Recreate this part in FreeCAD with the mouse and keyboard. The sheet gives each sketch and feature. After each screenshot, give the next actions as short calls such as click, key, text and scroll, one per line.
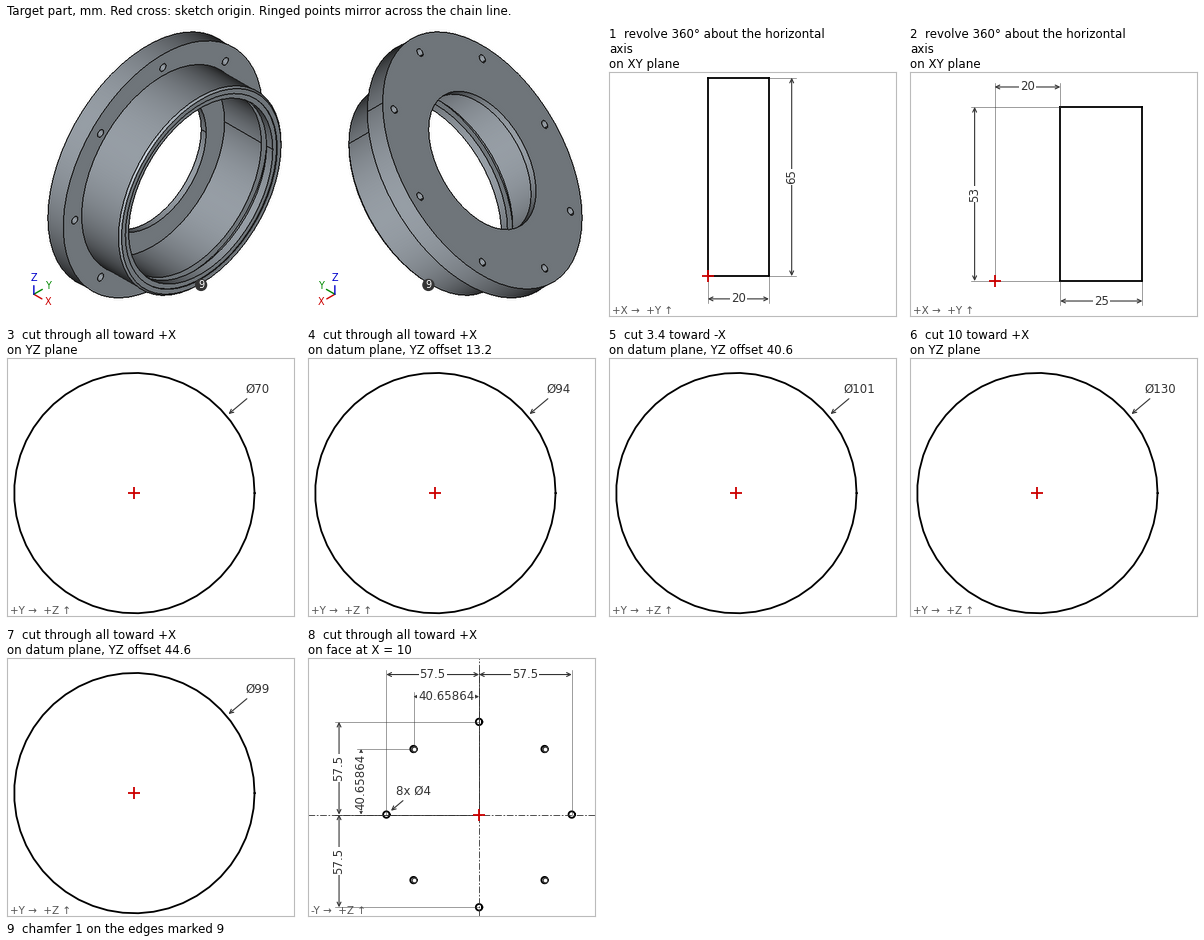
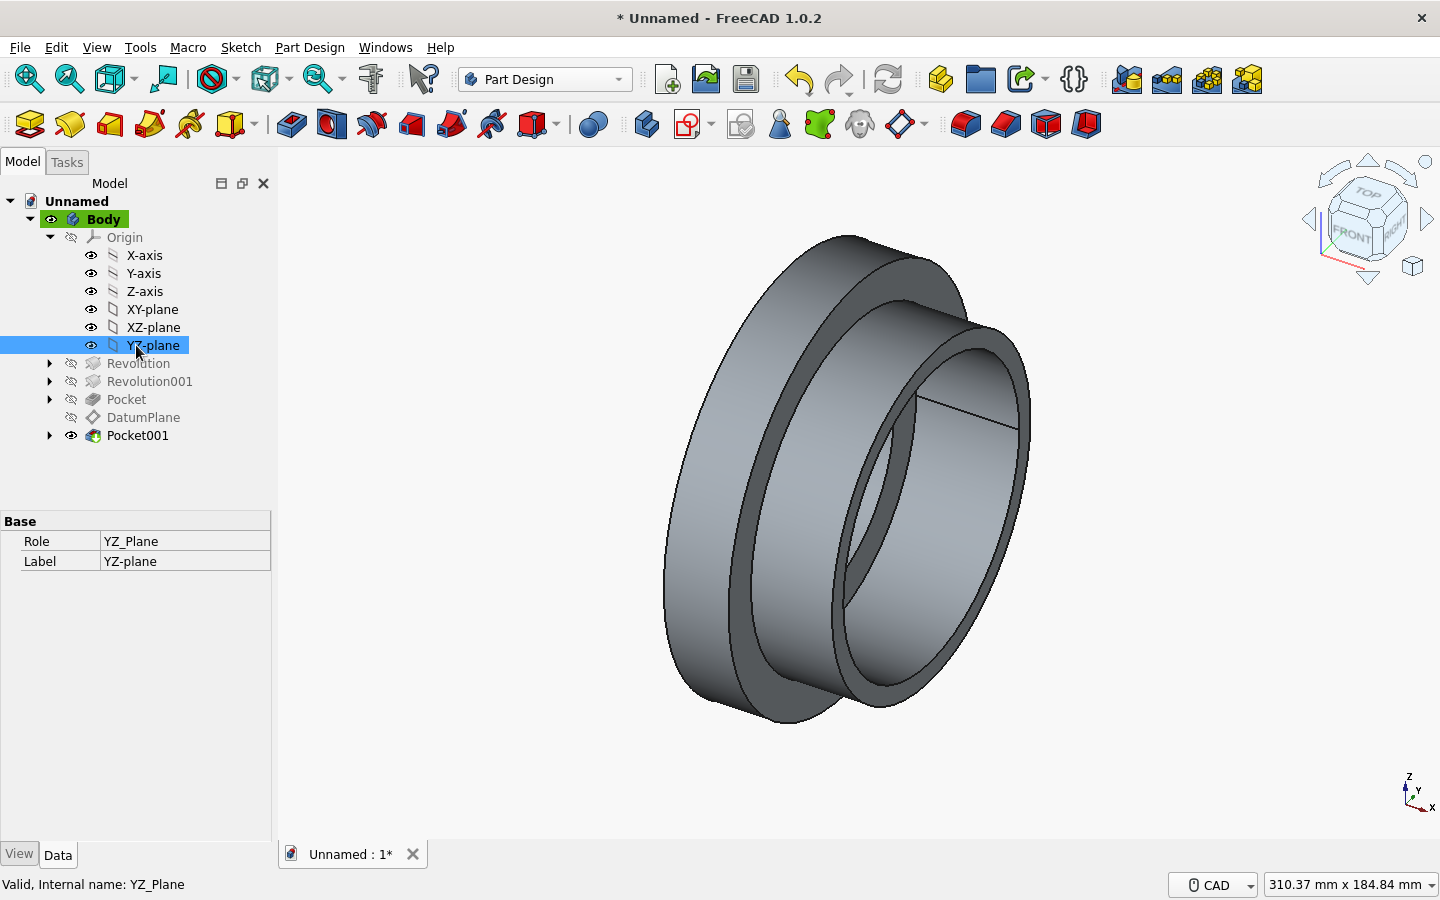
click(900, 124)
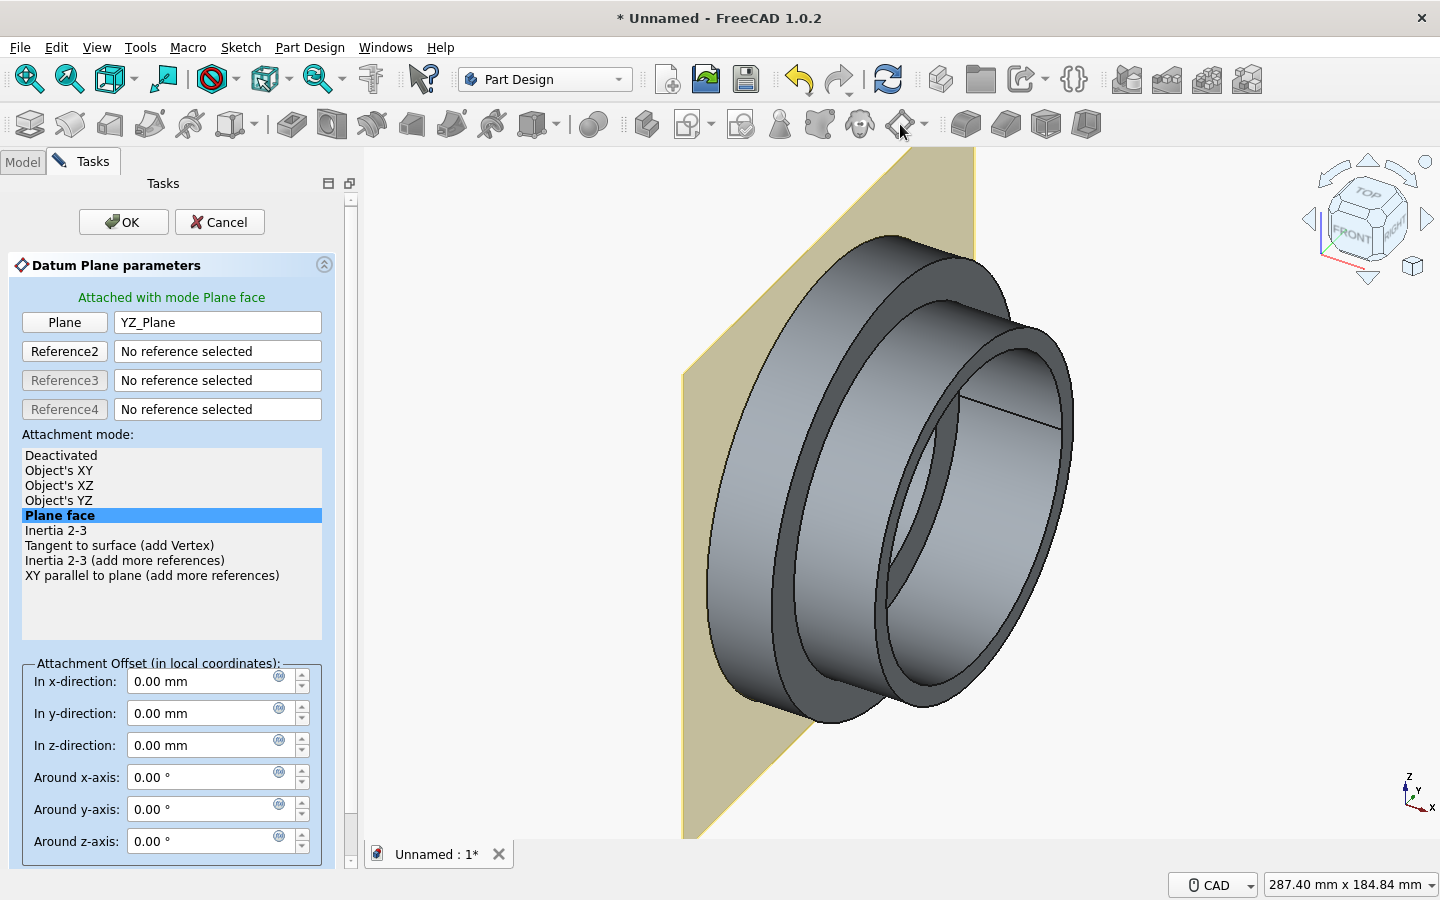
triple_click(210, 745)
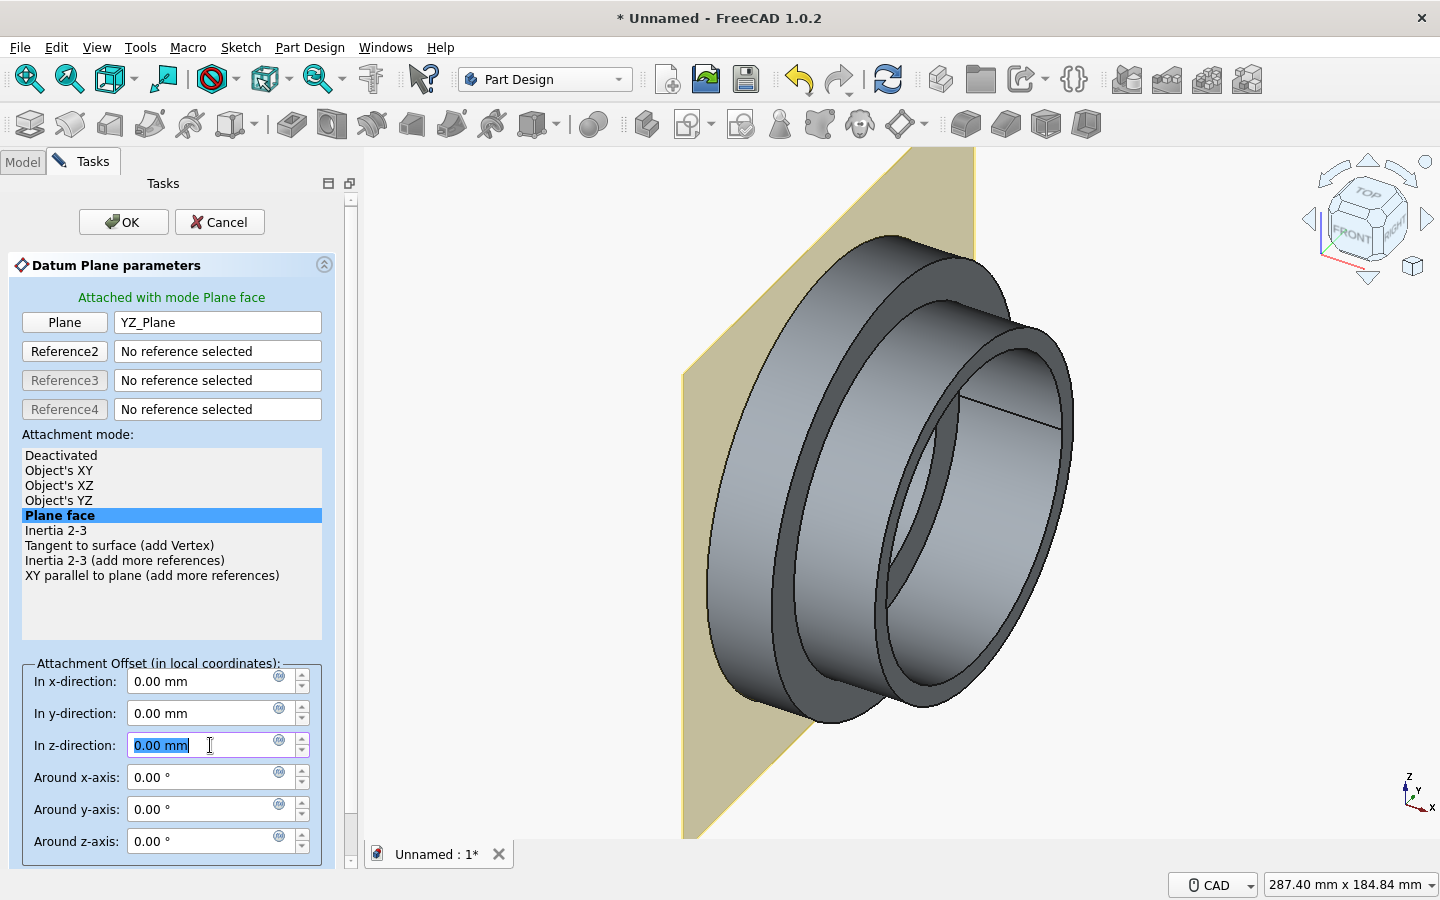
text(40.6)
key(Tab)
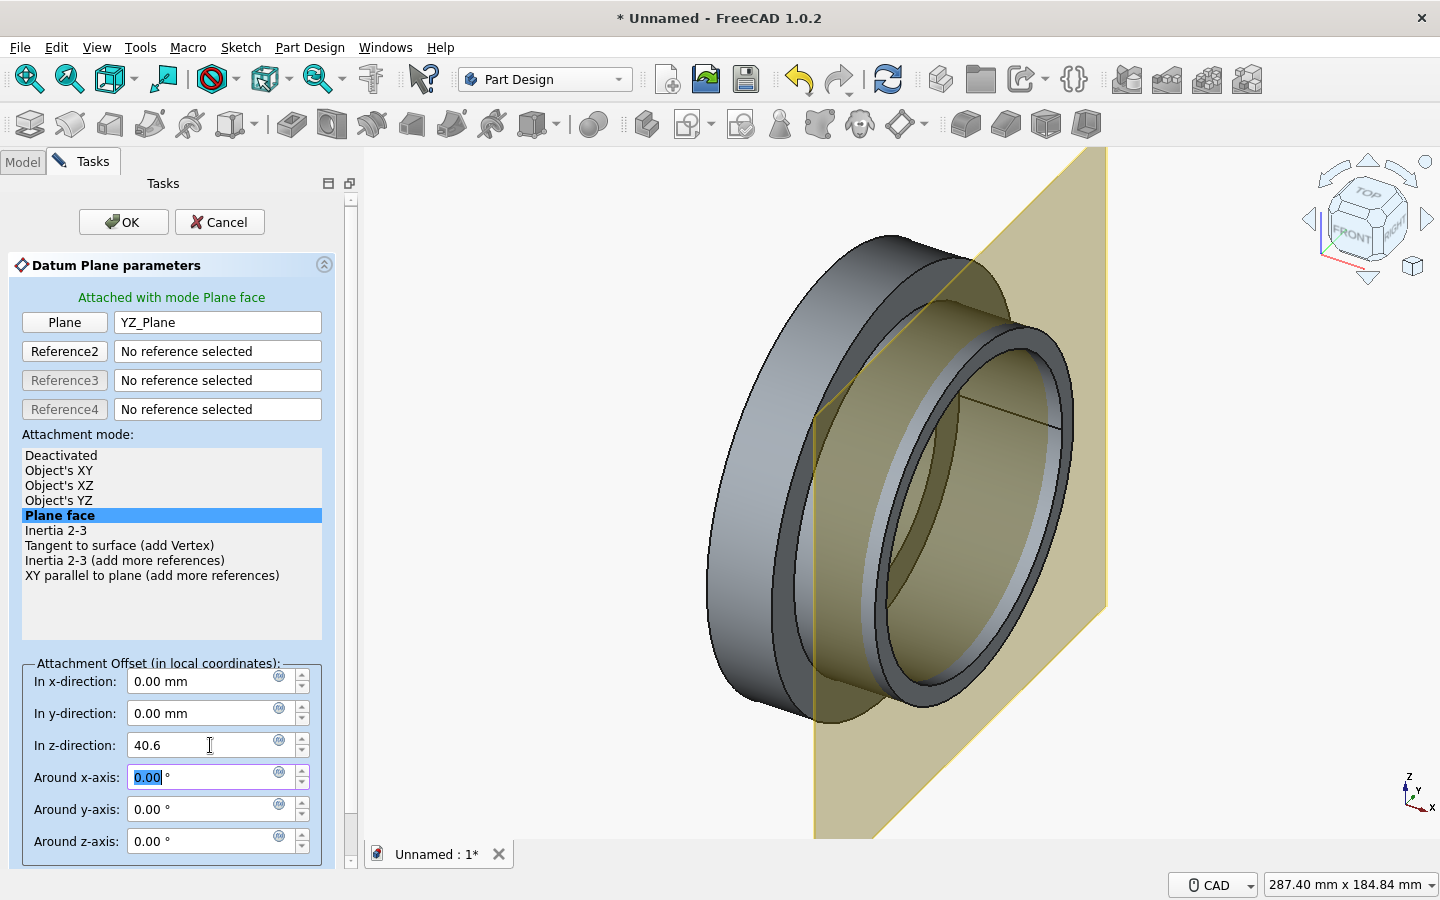
click(124, 222)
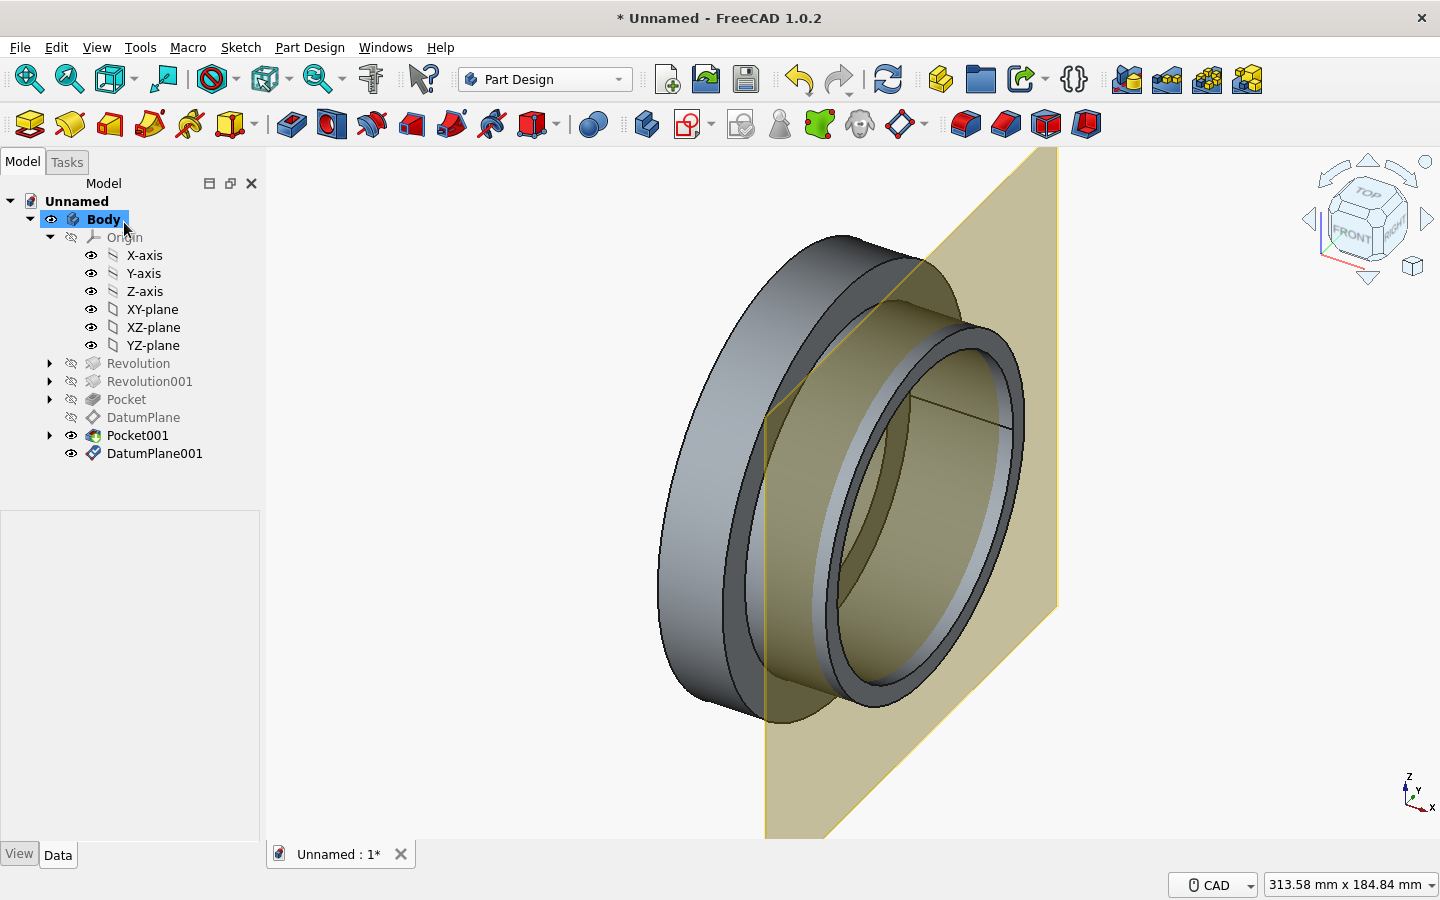
click(116, 453)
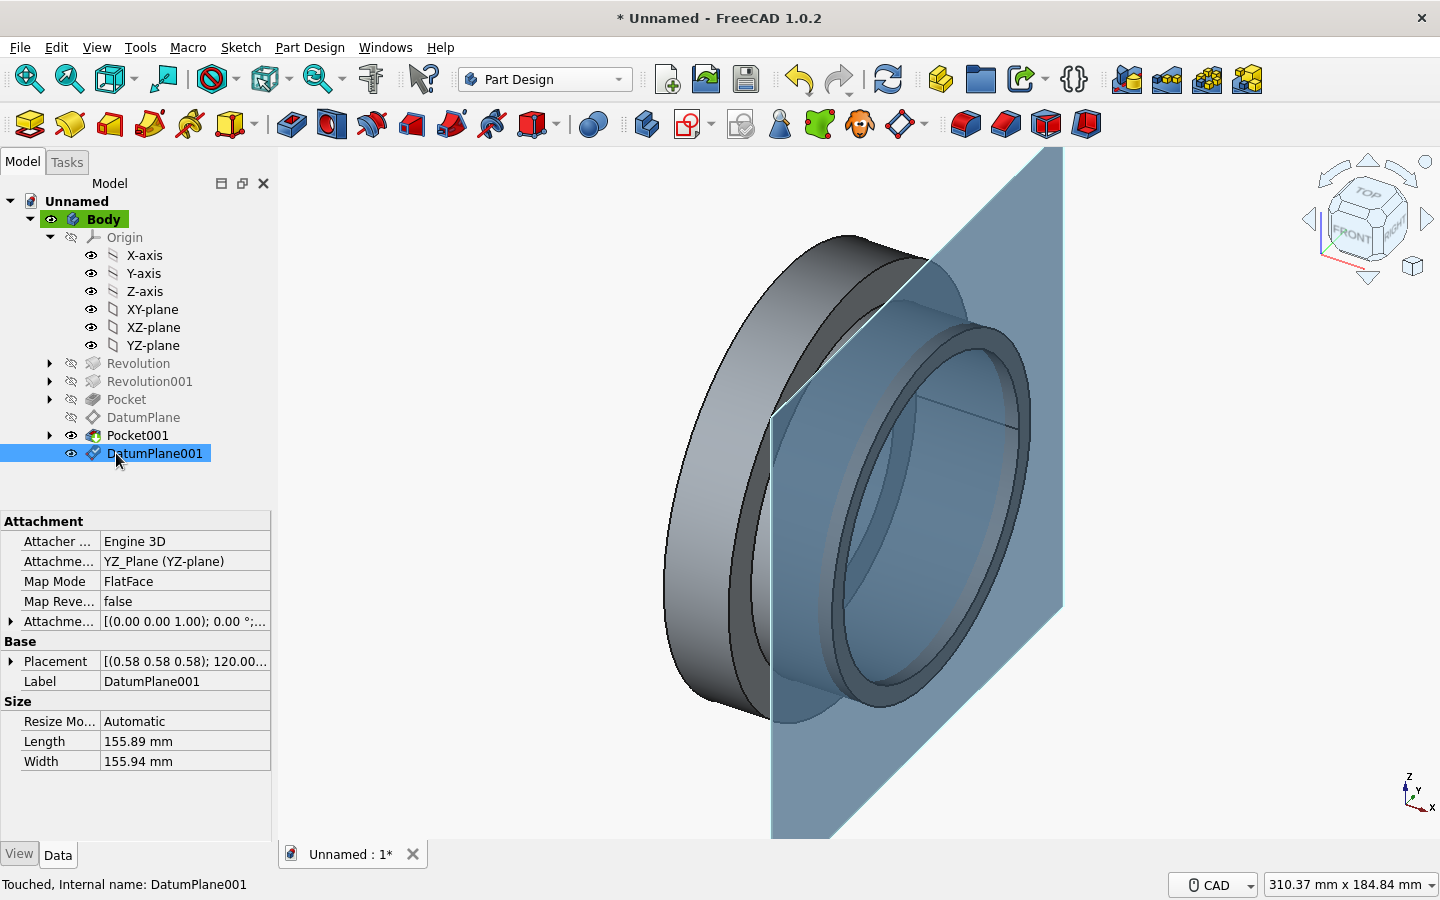
click(688, 124)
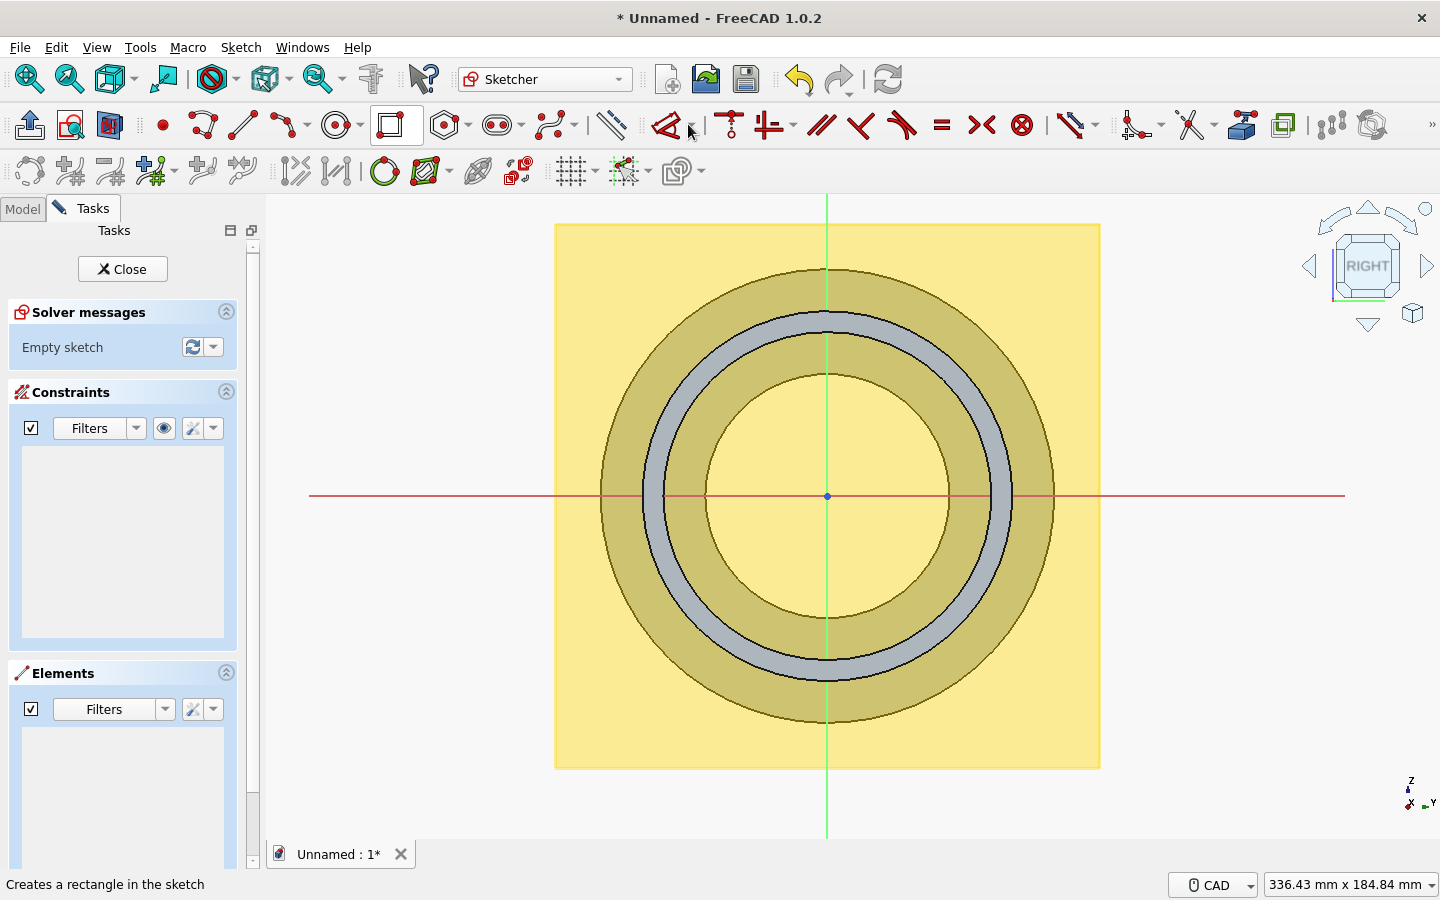
click(110, 126)